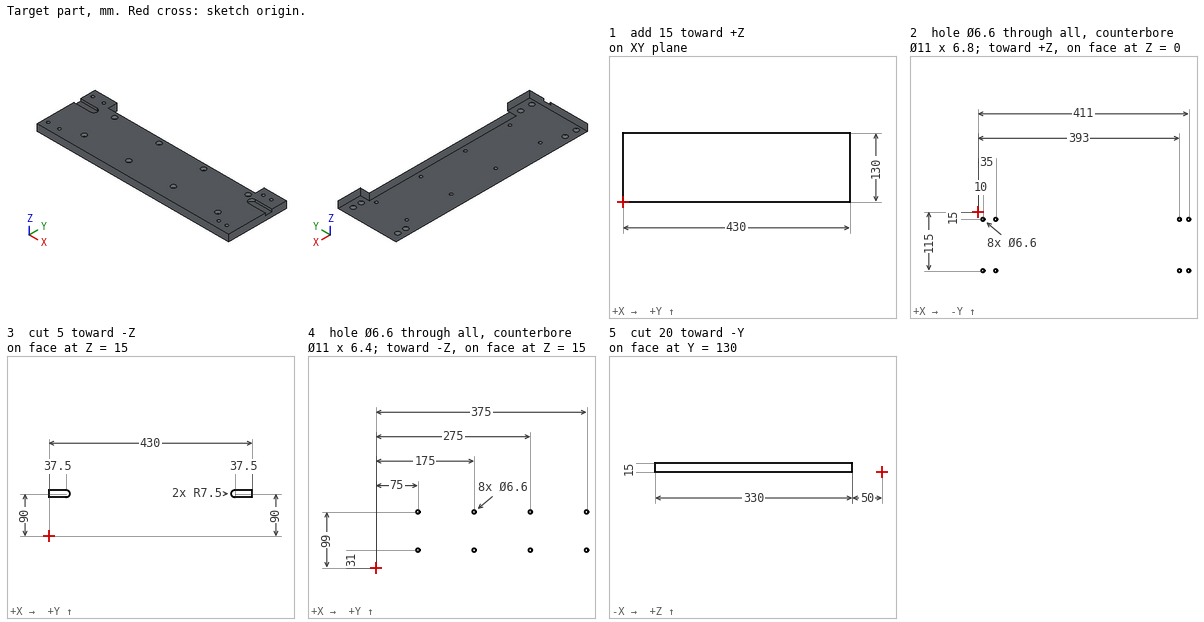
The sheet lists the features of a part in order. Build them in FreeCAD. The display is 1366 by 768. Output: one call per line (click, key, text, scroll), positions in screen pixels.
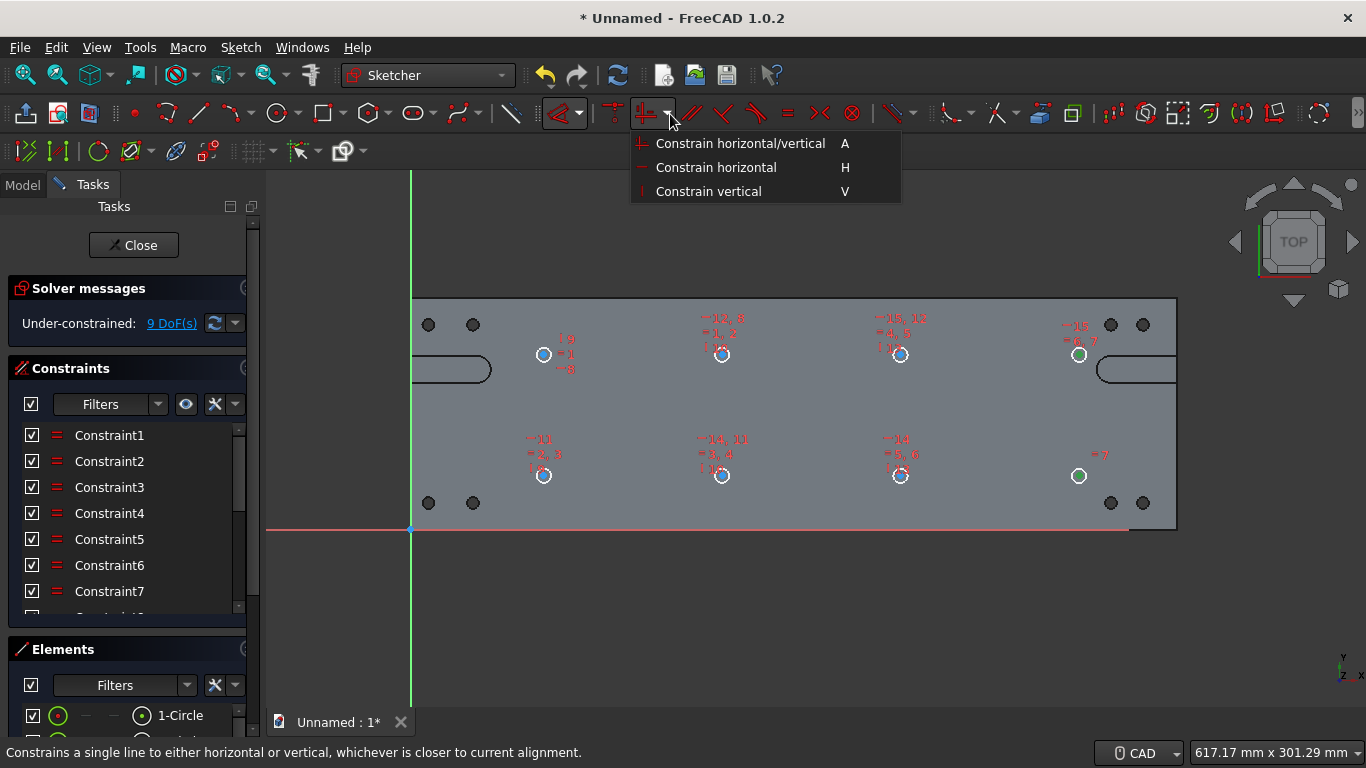
click(766, 191)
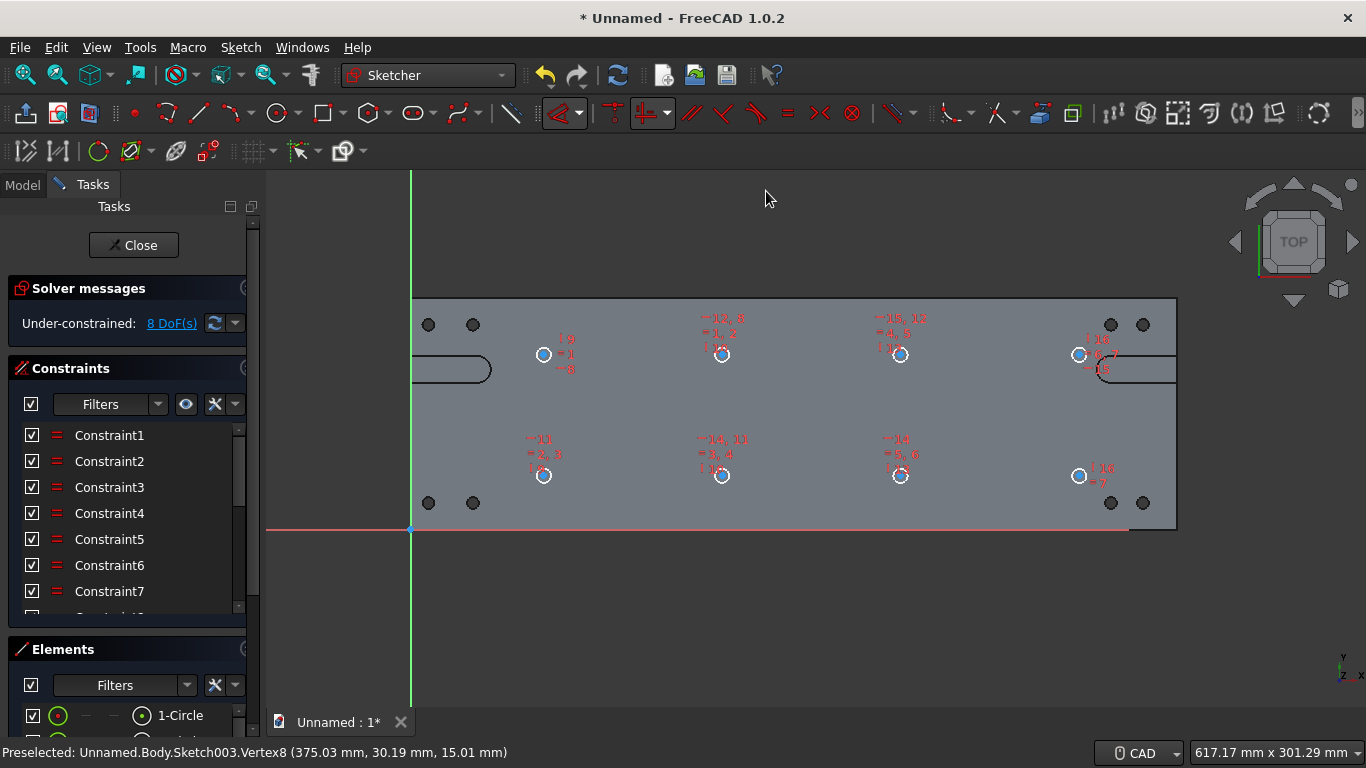
click(900, 476)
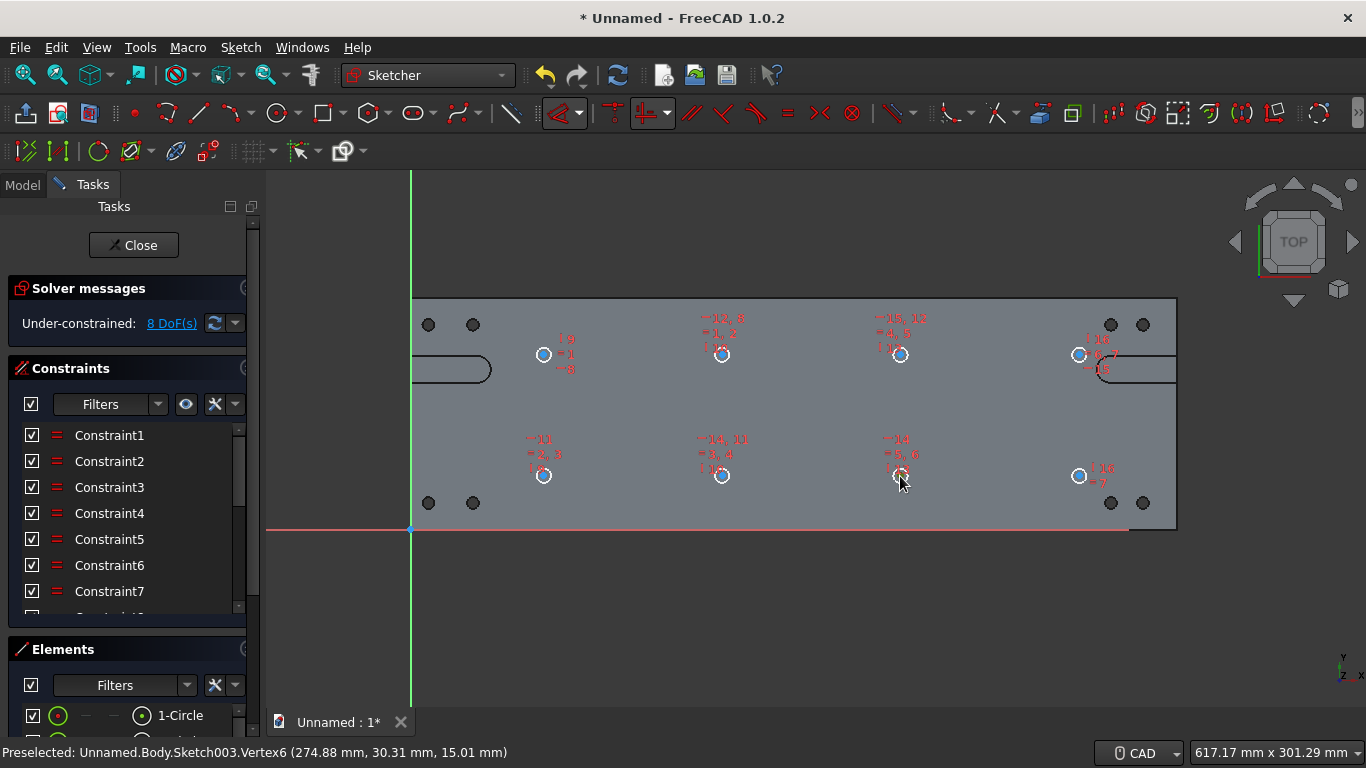
click(1079, 476)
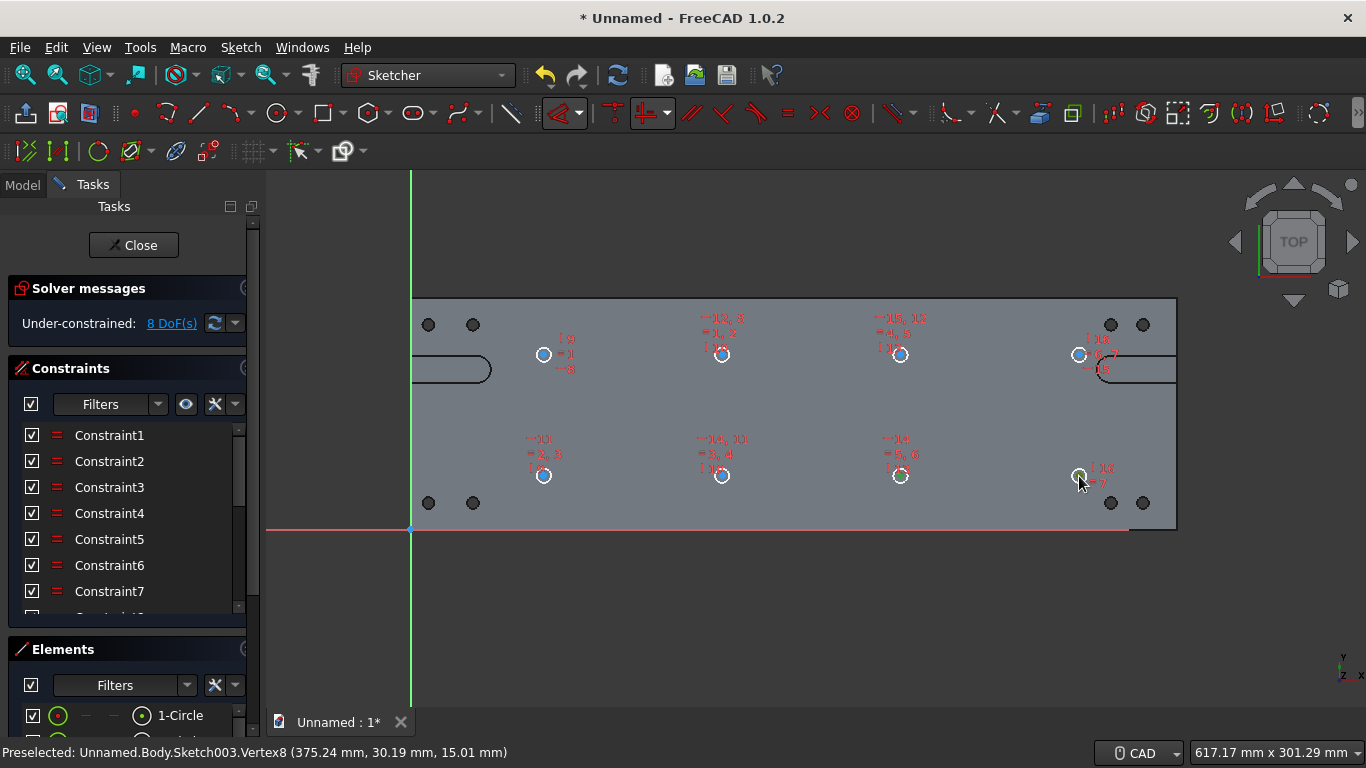
key(h)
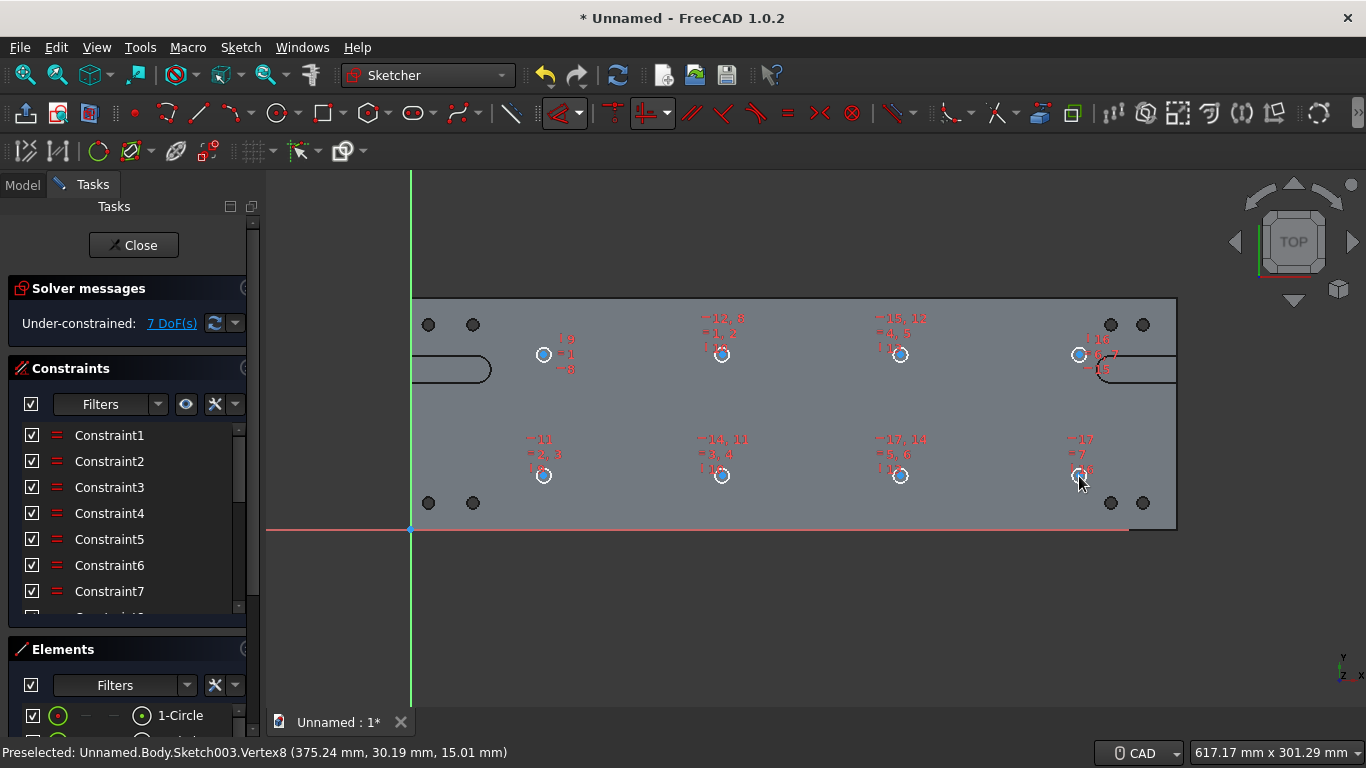
scroll(544, 362, up, 7)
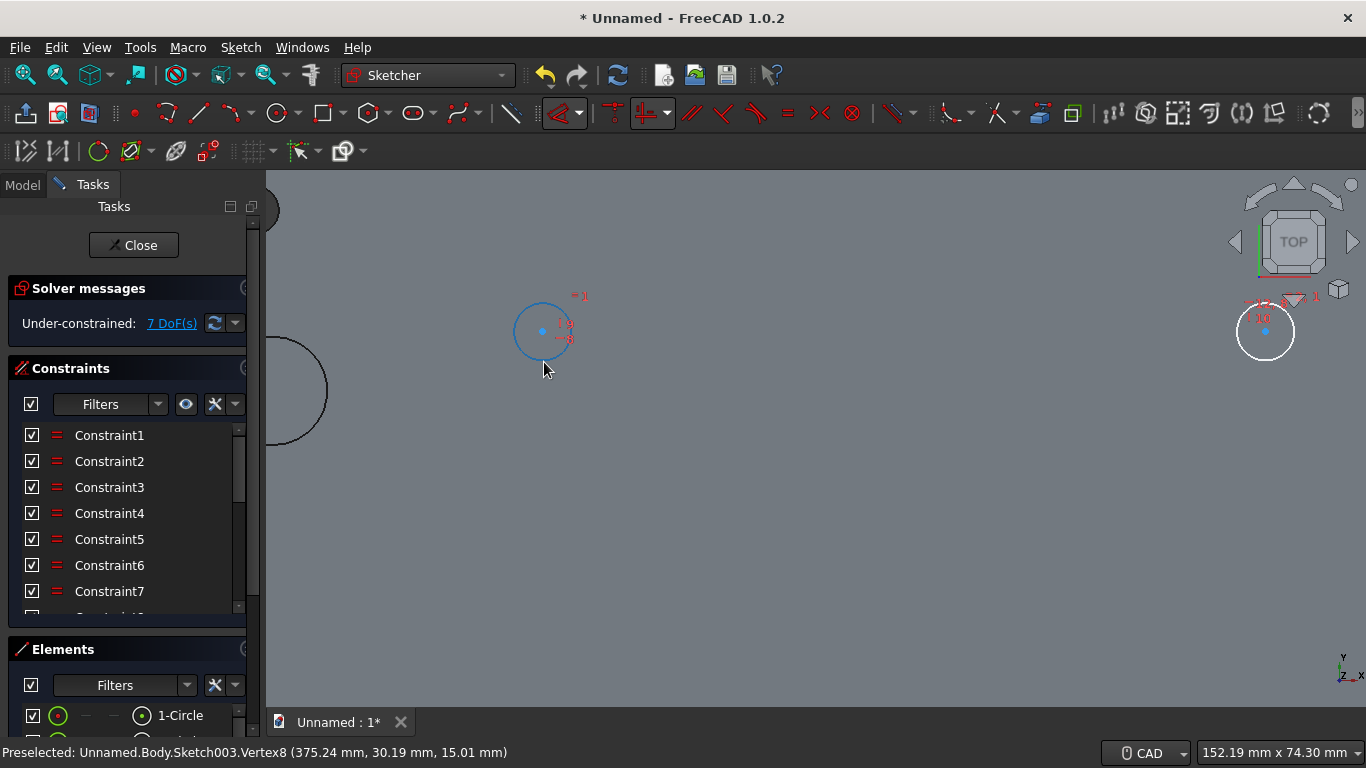
click(542, 360)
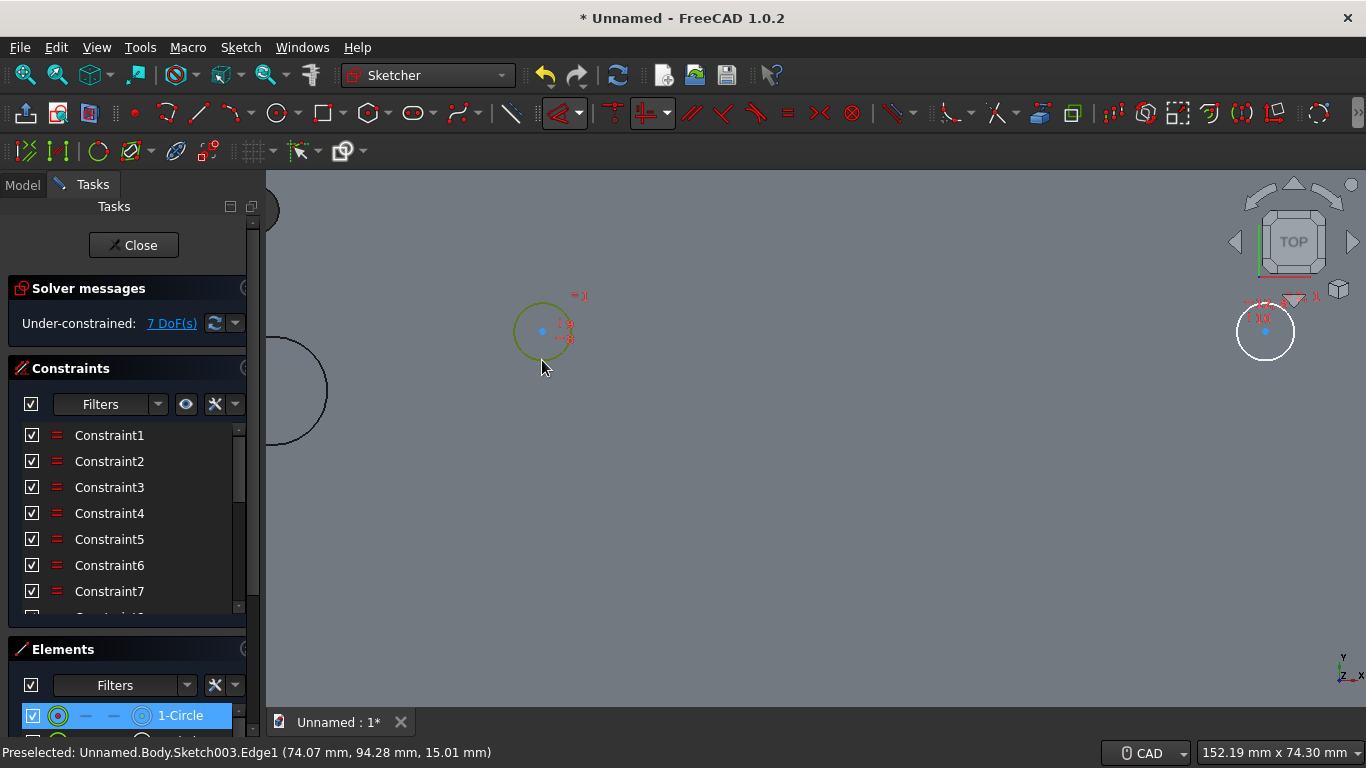
key(k)
key(o)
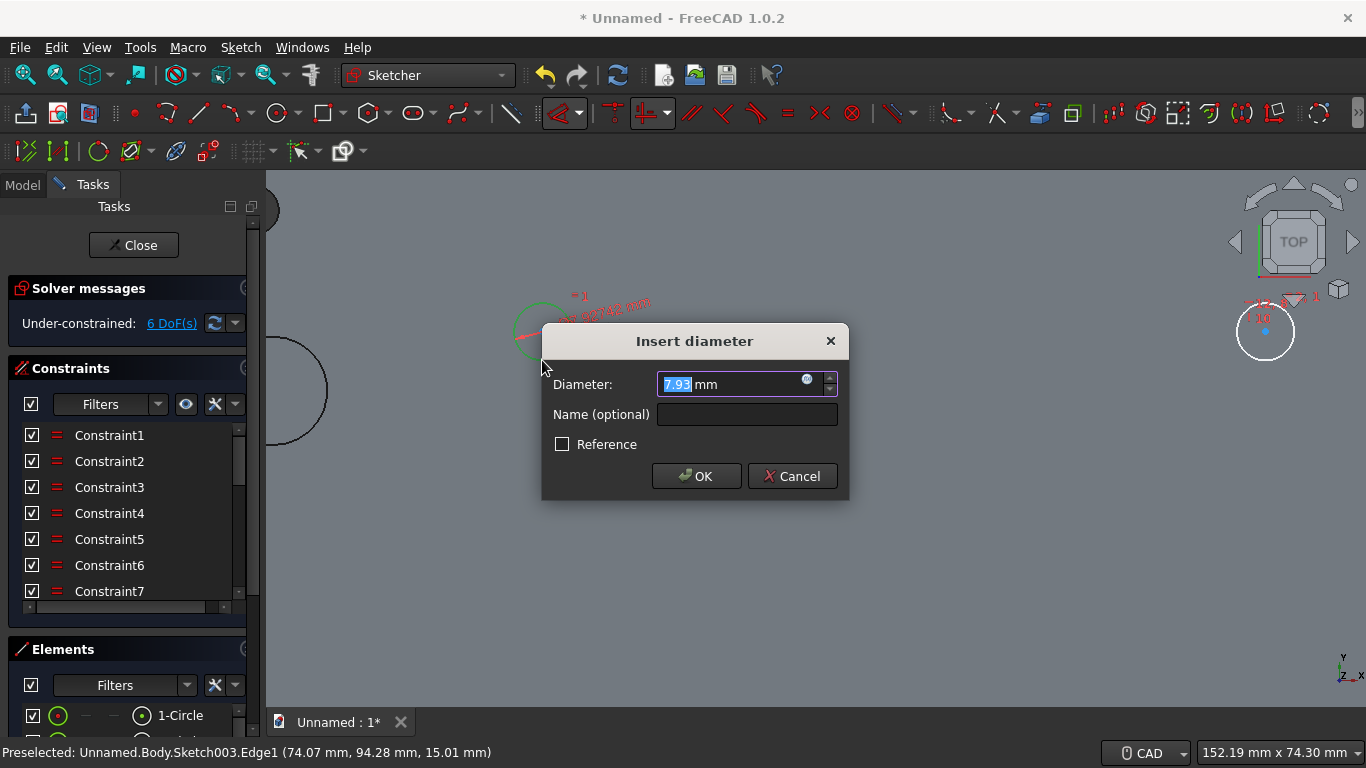
text(6.6)
key(Return)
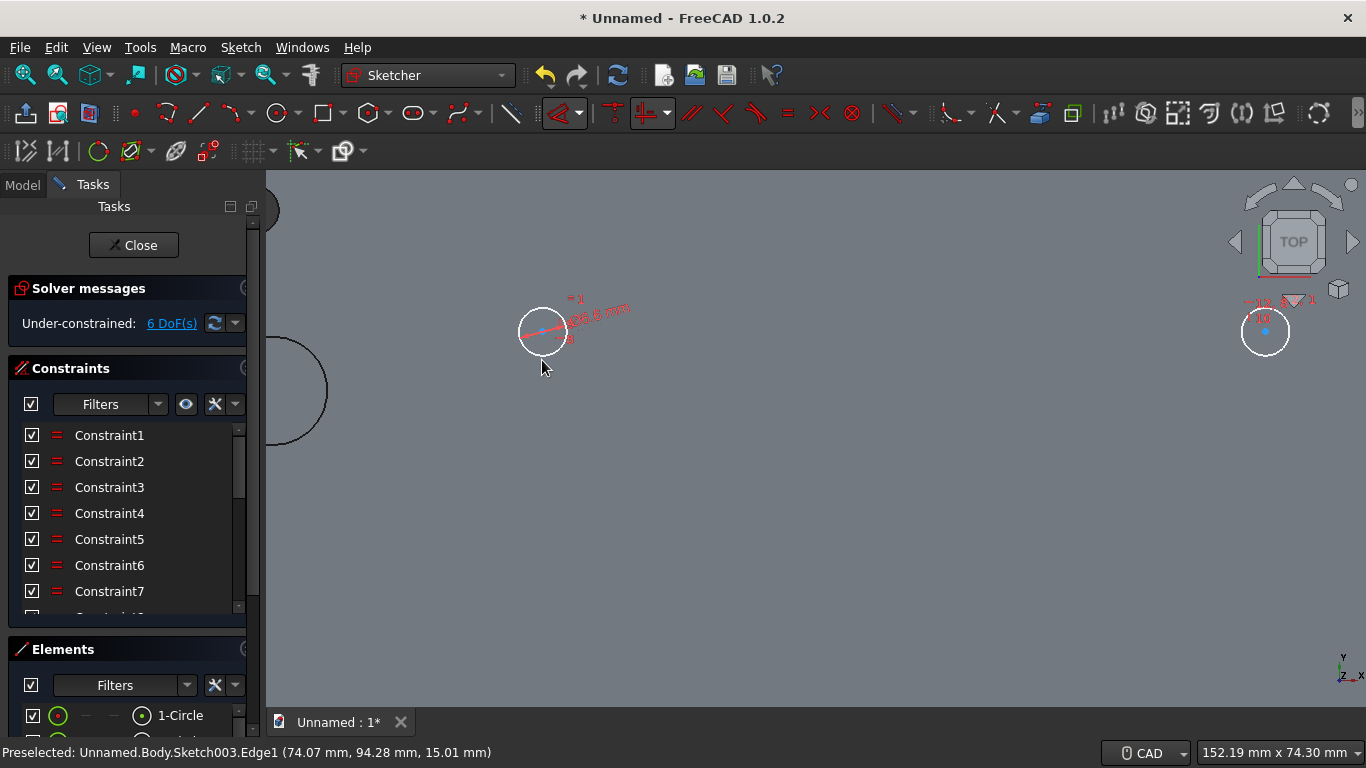
scroll(544, 362, down, 7)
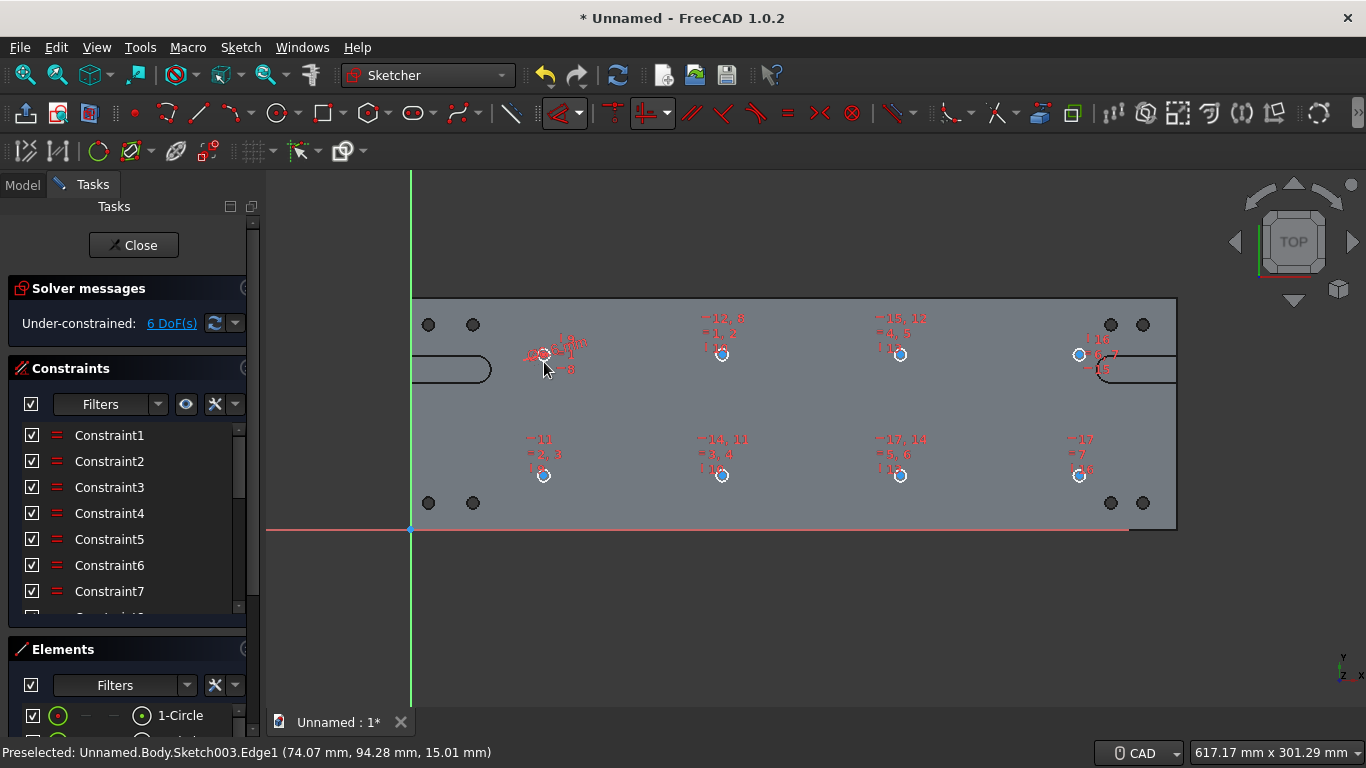
click(544, 355)